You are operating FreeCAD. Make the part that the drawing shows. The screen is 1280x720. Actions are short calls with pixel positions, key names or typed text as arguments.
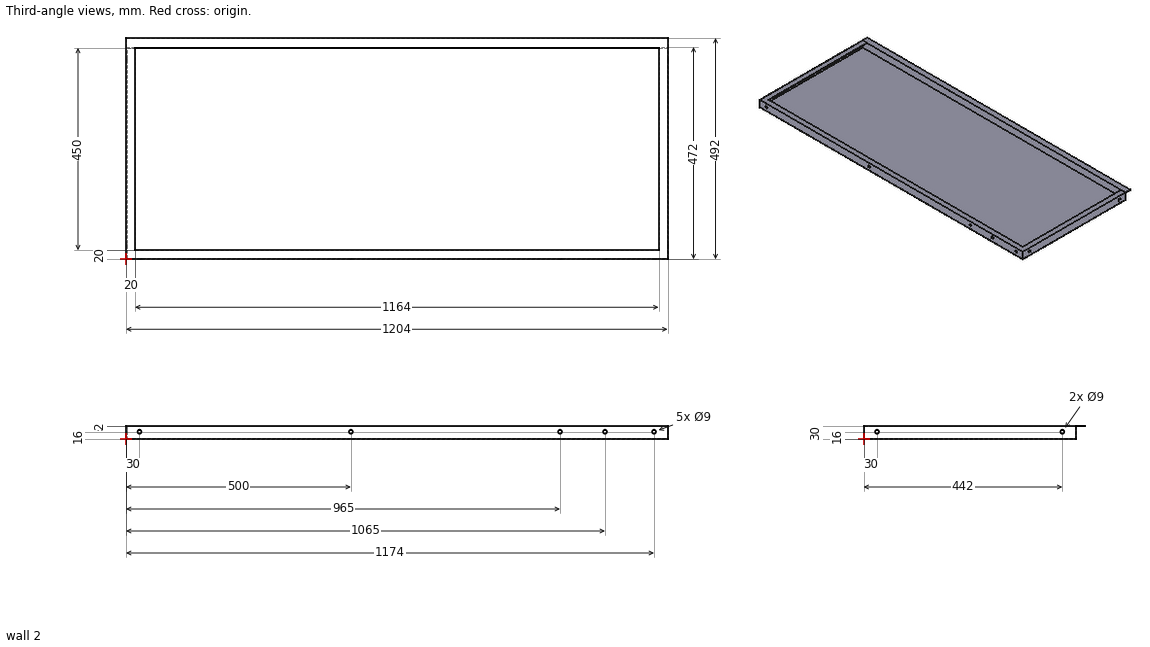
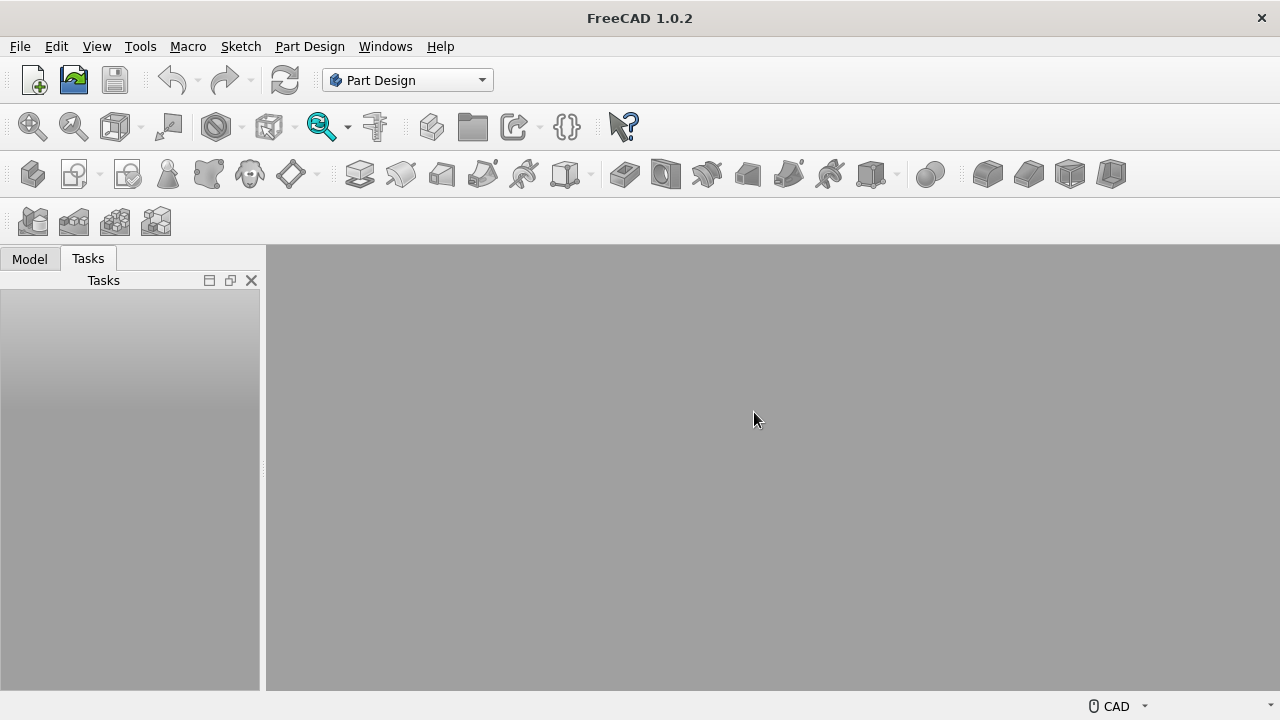
key(ctrl+n)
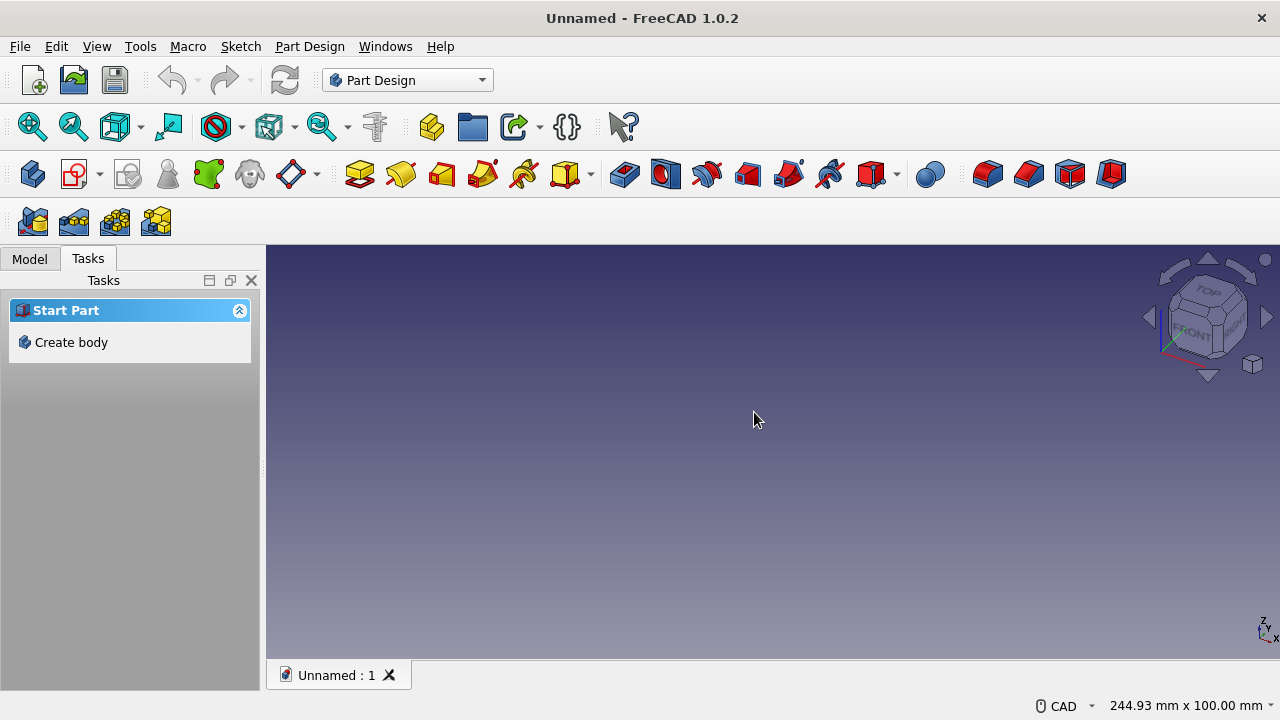
click(74, 174)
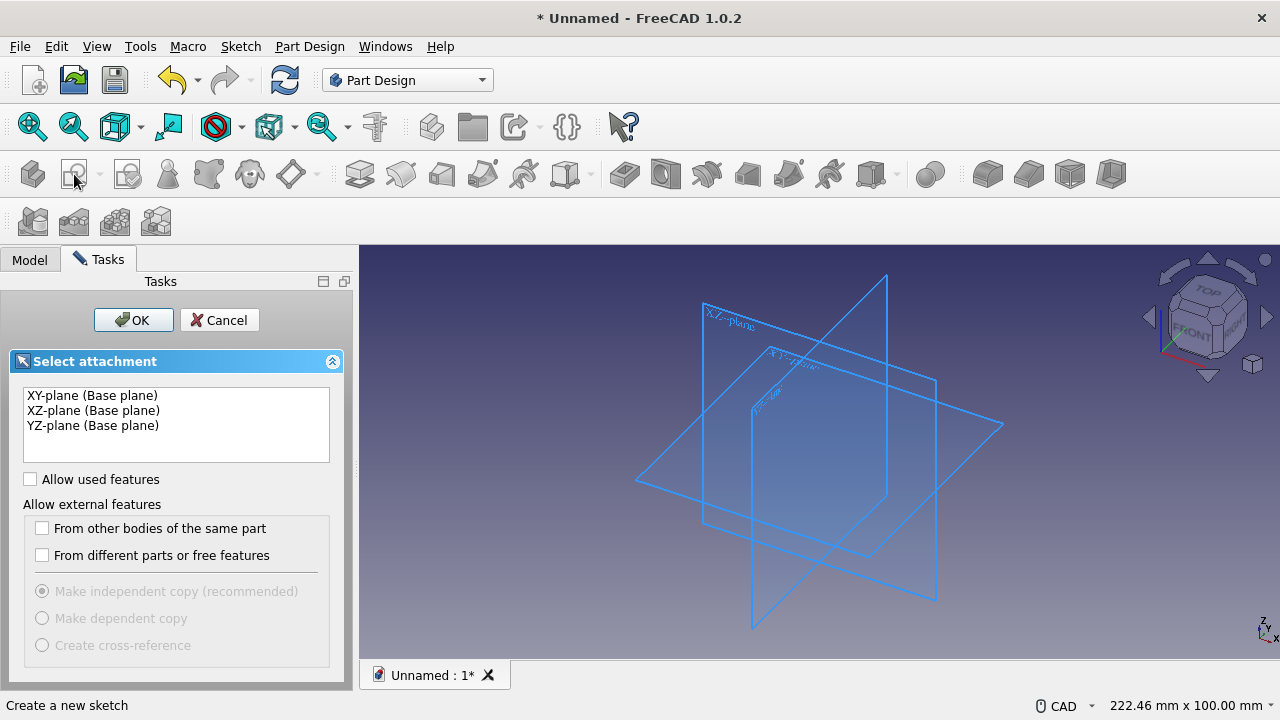
click(84, 396)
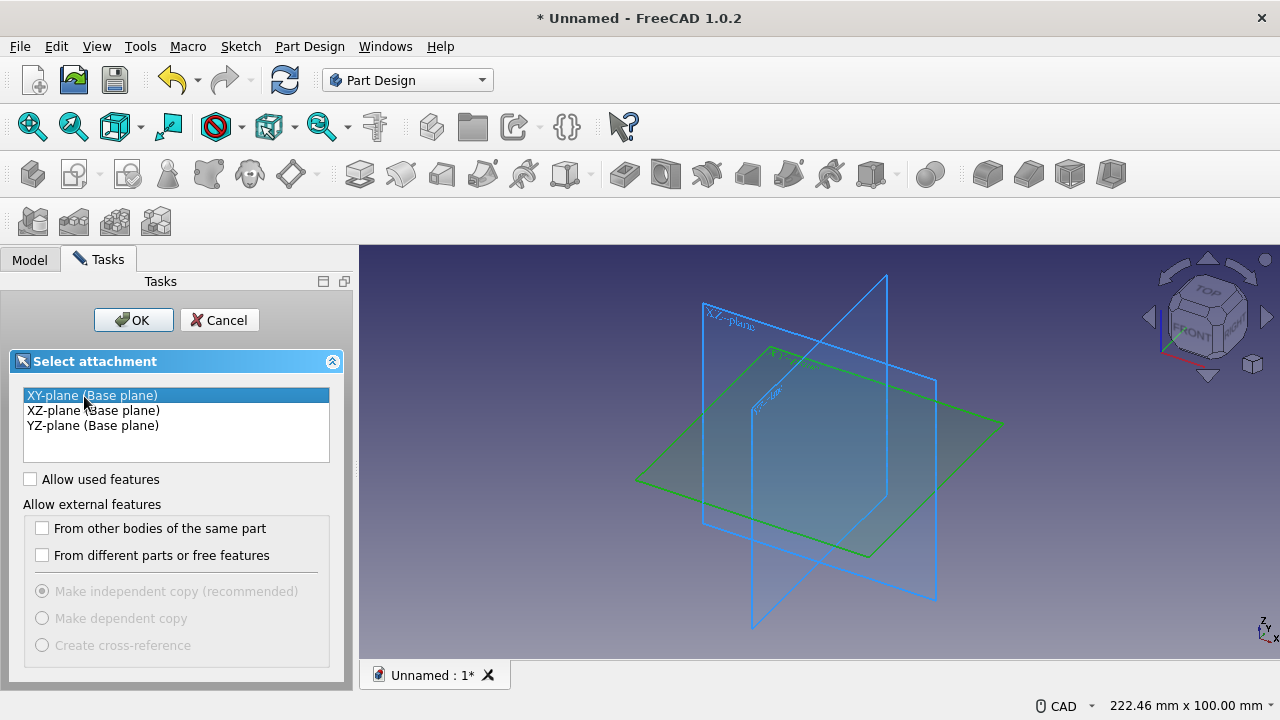
click(134, 320)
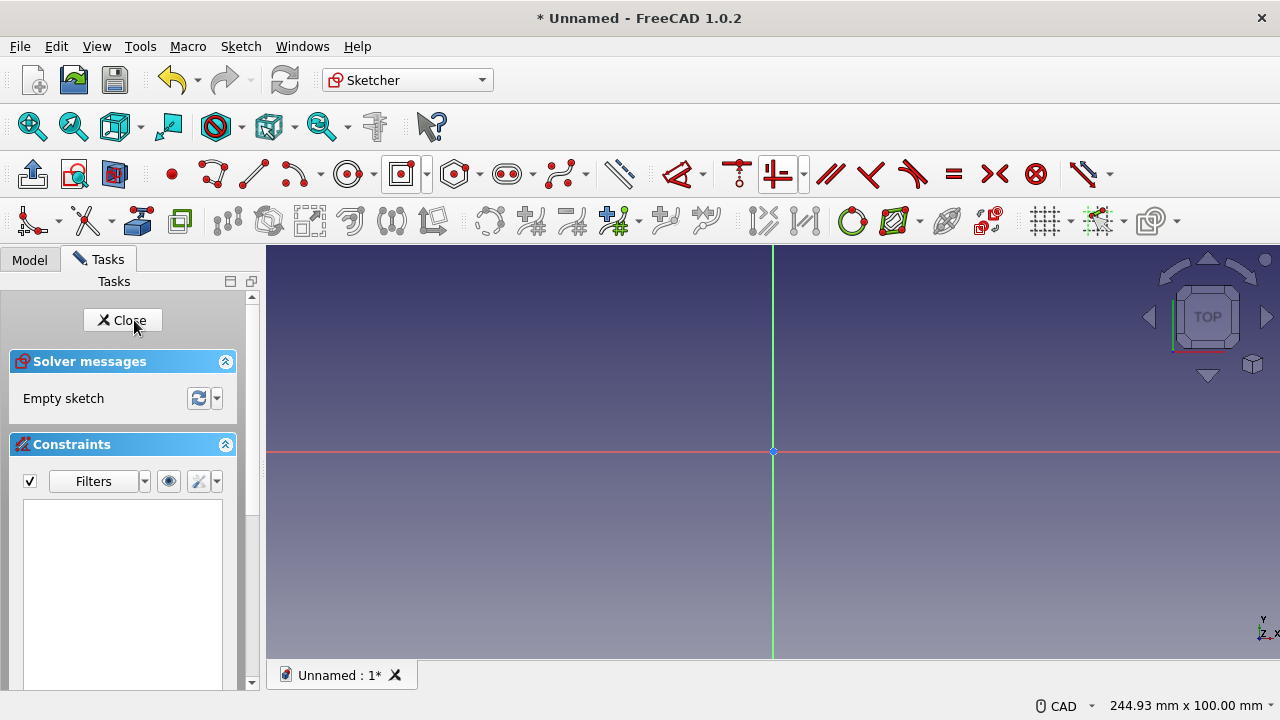
scroll(385, 574, down, 11)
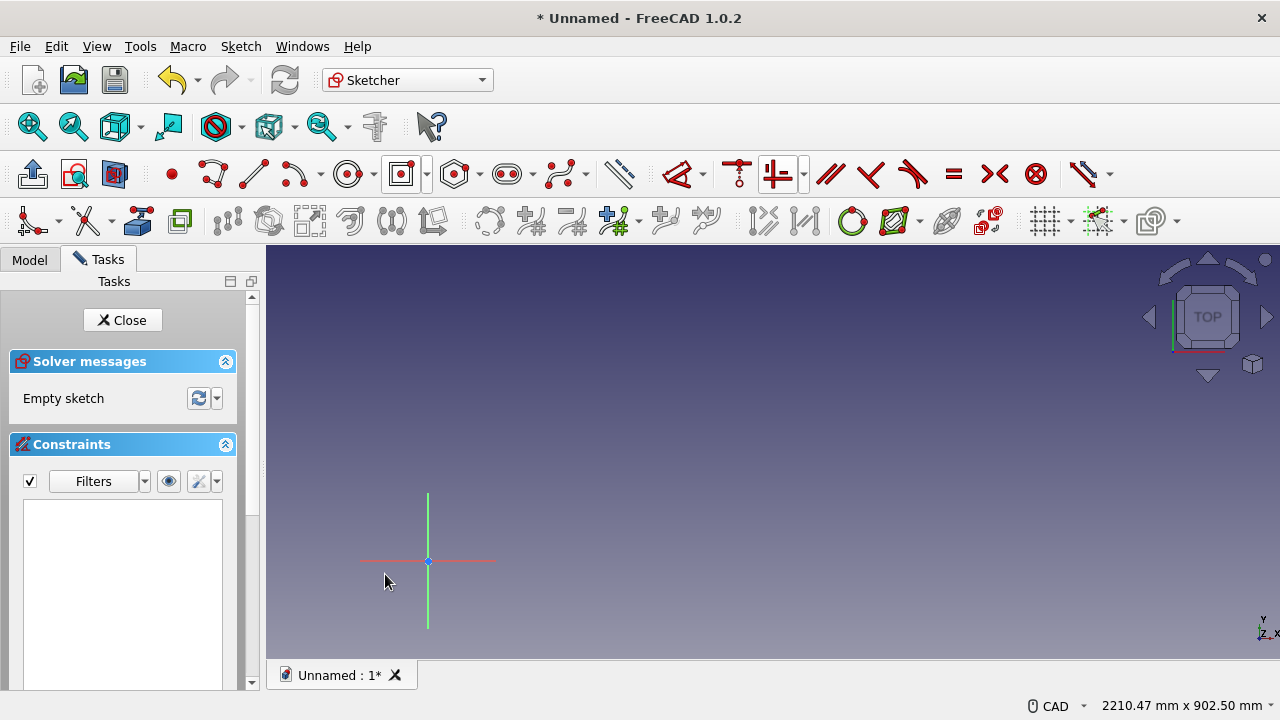
click(426, 174)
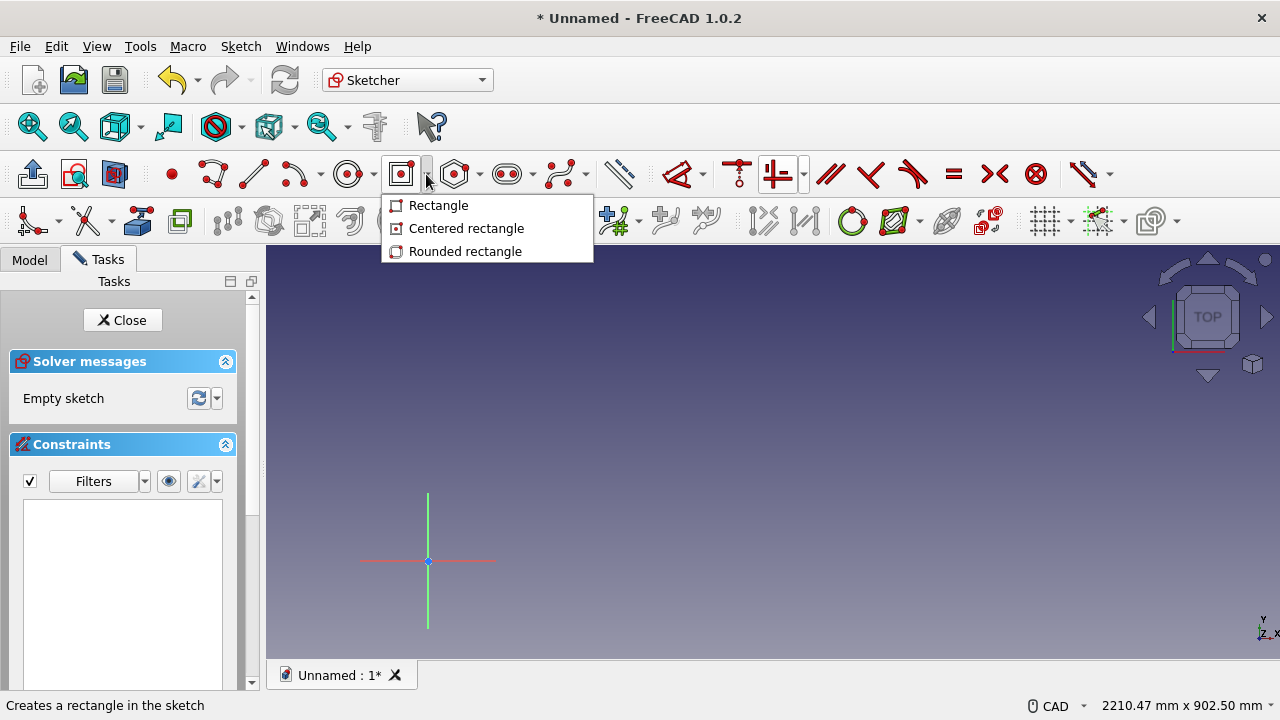
click(488, 206)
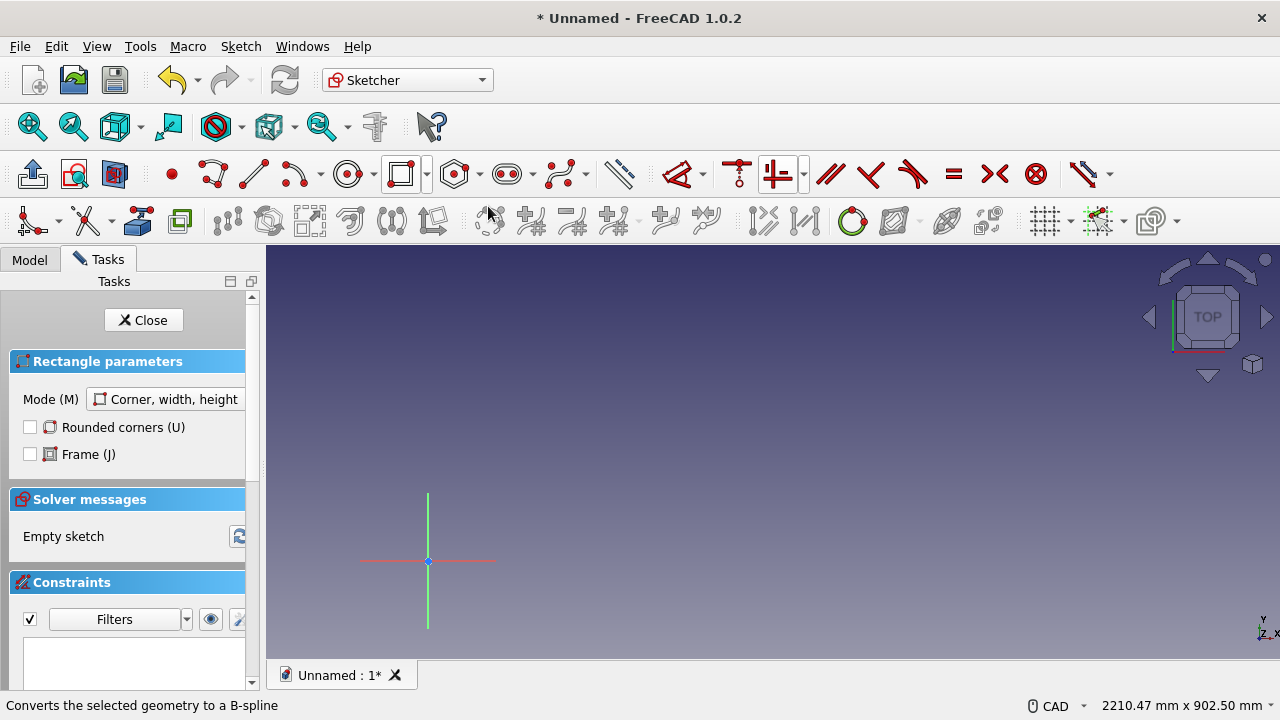
click(428, 561)
click(980, 345)
key(Escape)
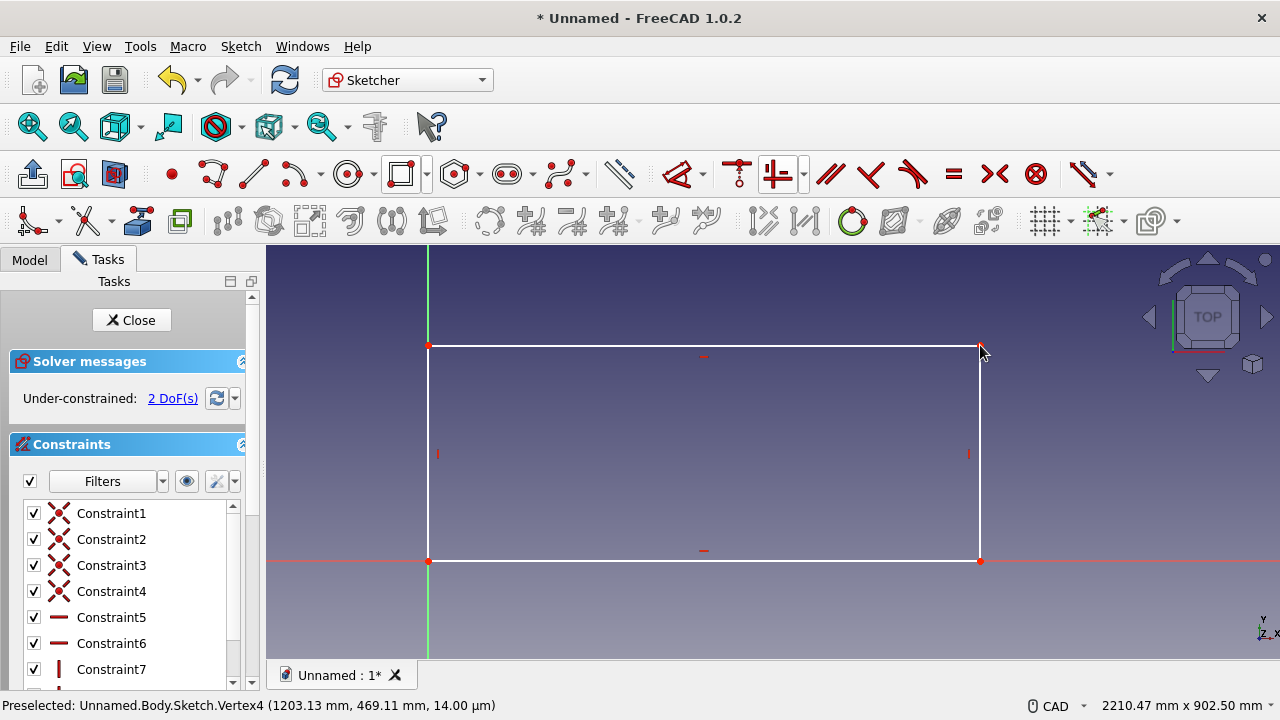
key(d)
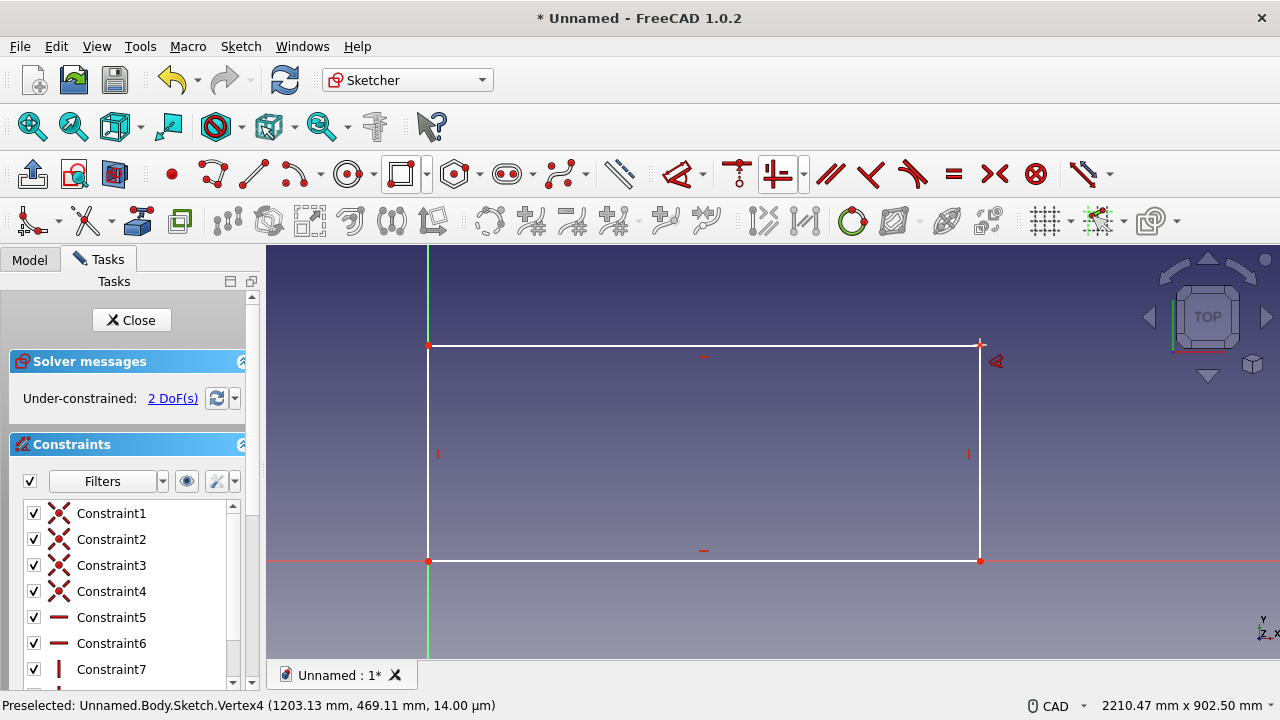
click(980, 497)
click(1014, 454)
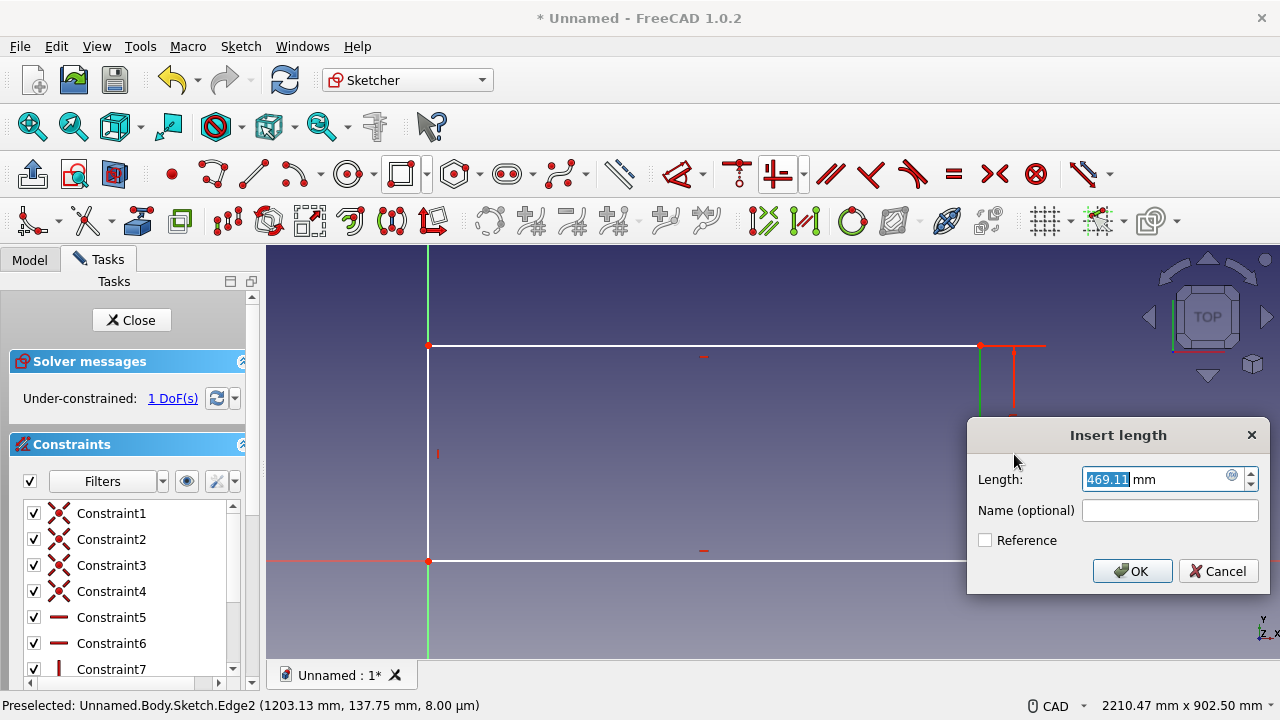
text(472)
key(Return)